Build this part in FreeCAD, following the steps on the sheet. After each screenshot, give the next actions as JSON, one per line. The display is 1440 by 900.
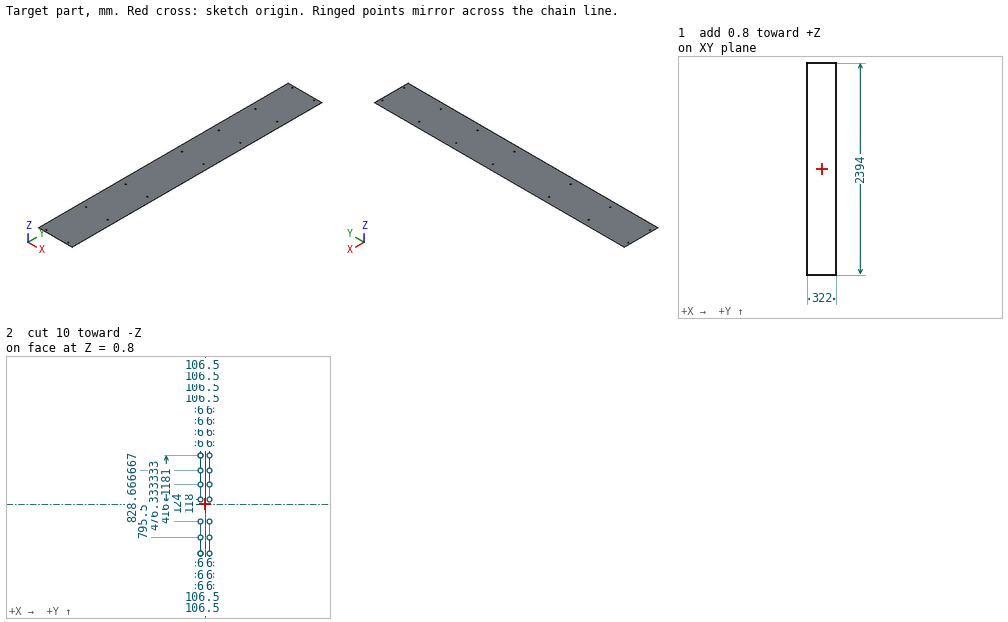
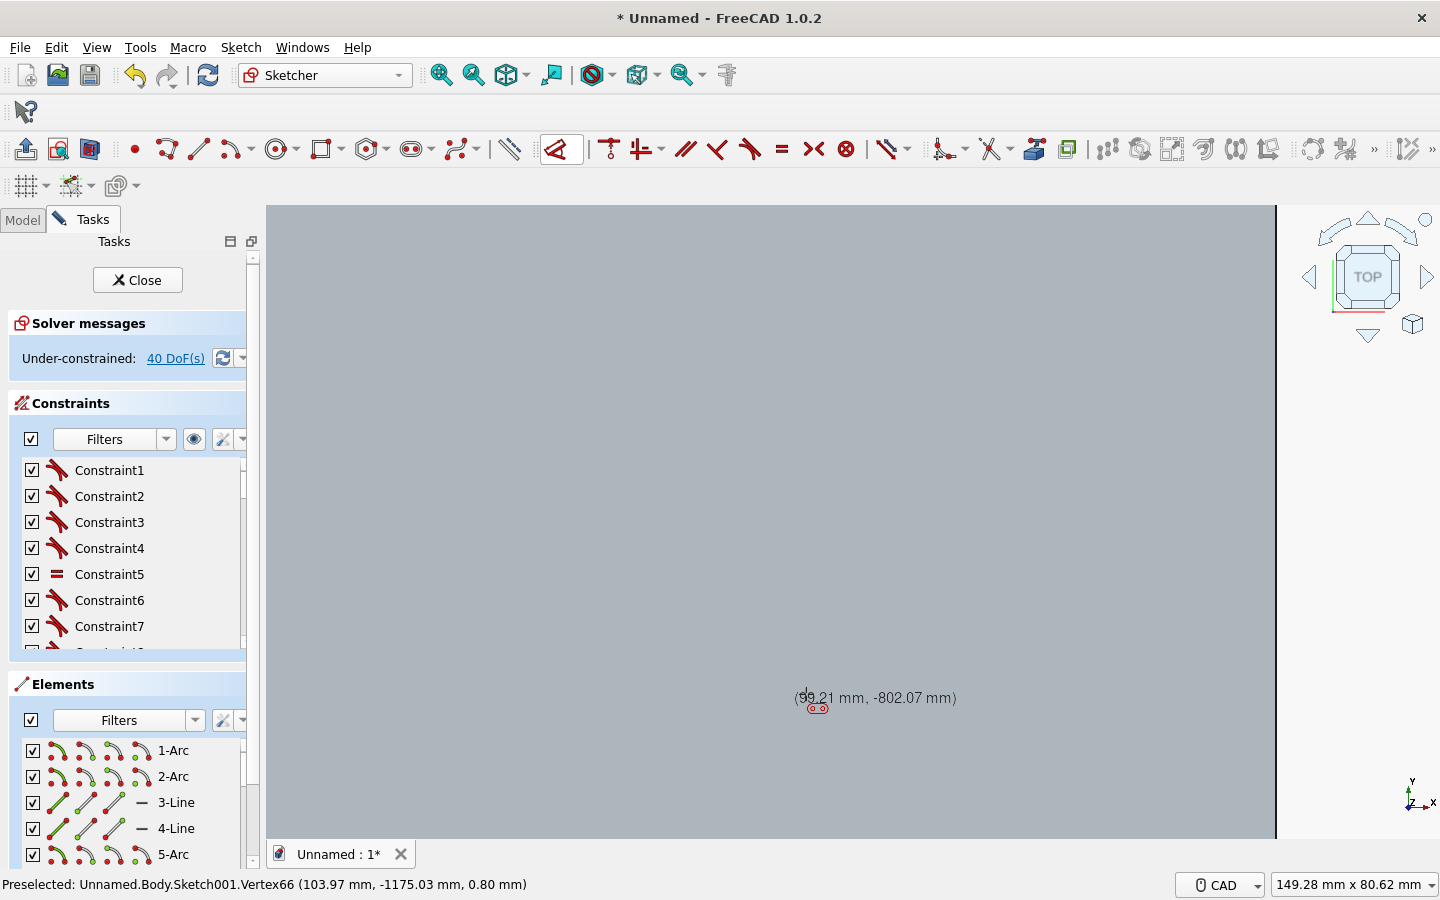
{"action": "scroll", "coordinate": [806, 694], "scroll_direction": "down", "scroll_amount": 18}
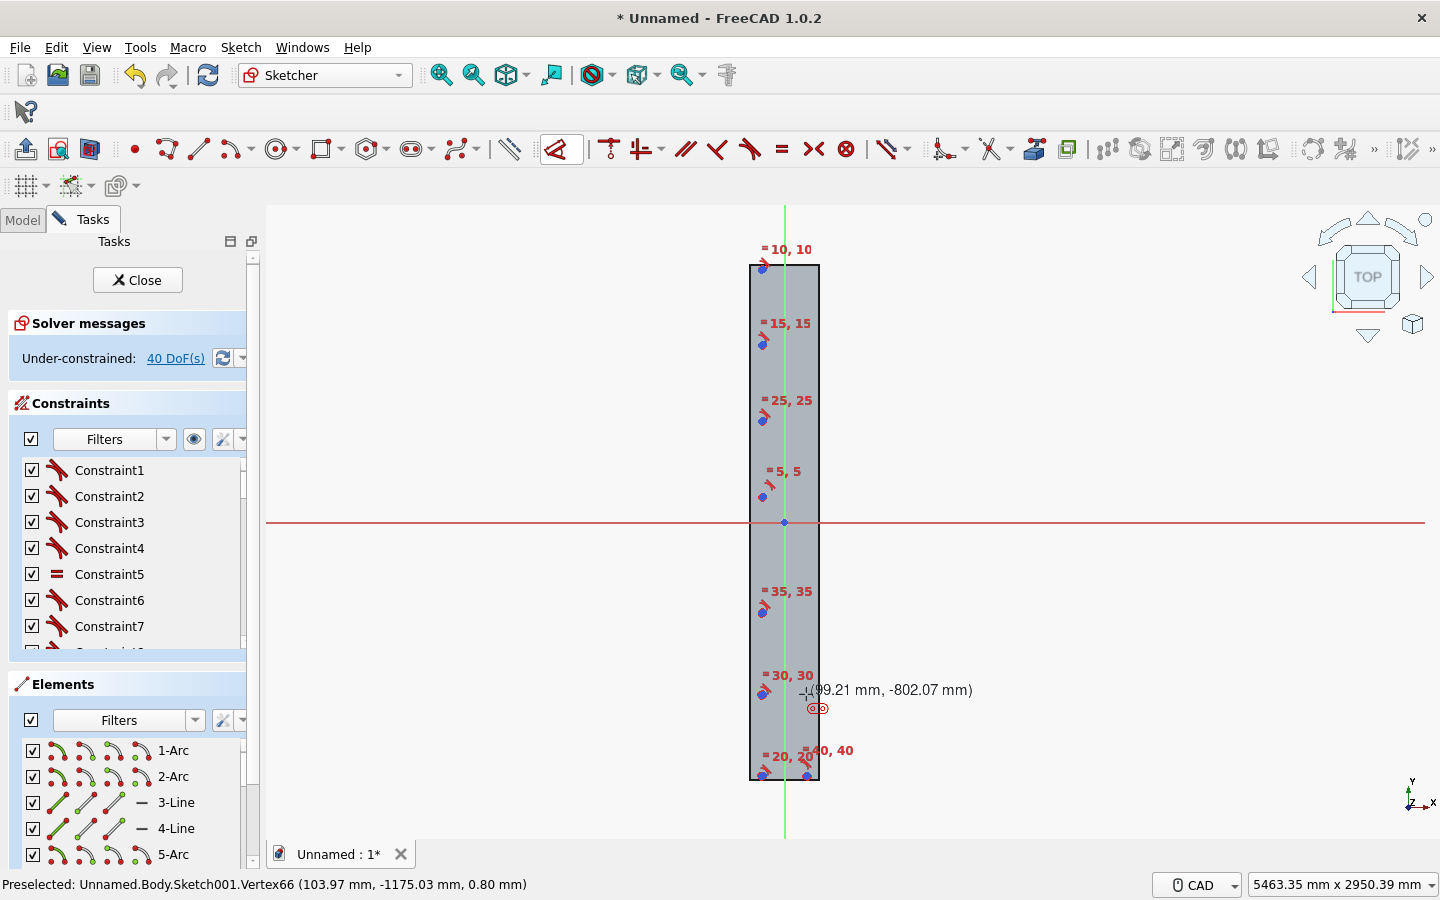
{"action": "left_click", "coordinate": [806, 694]}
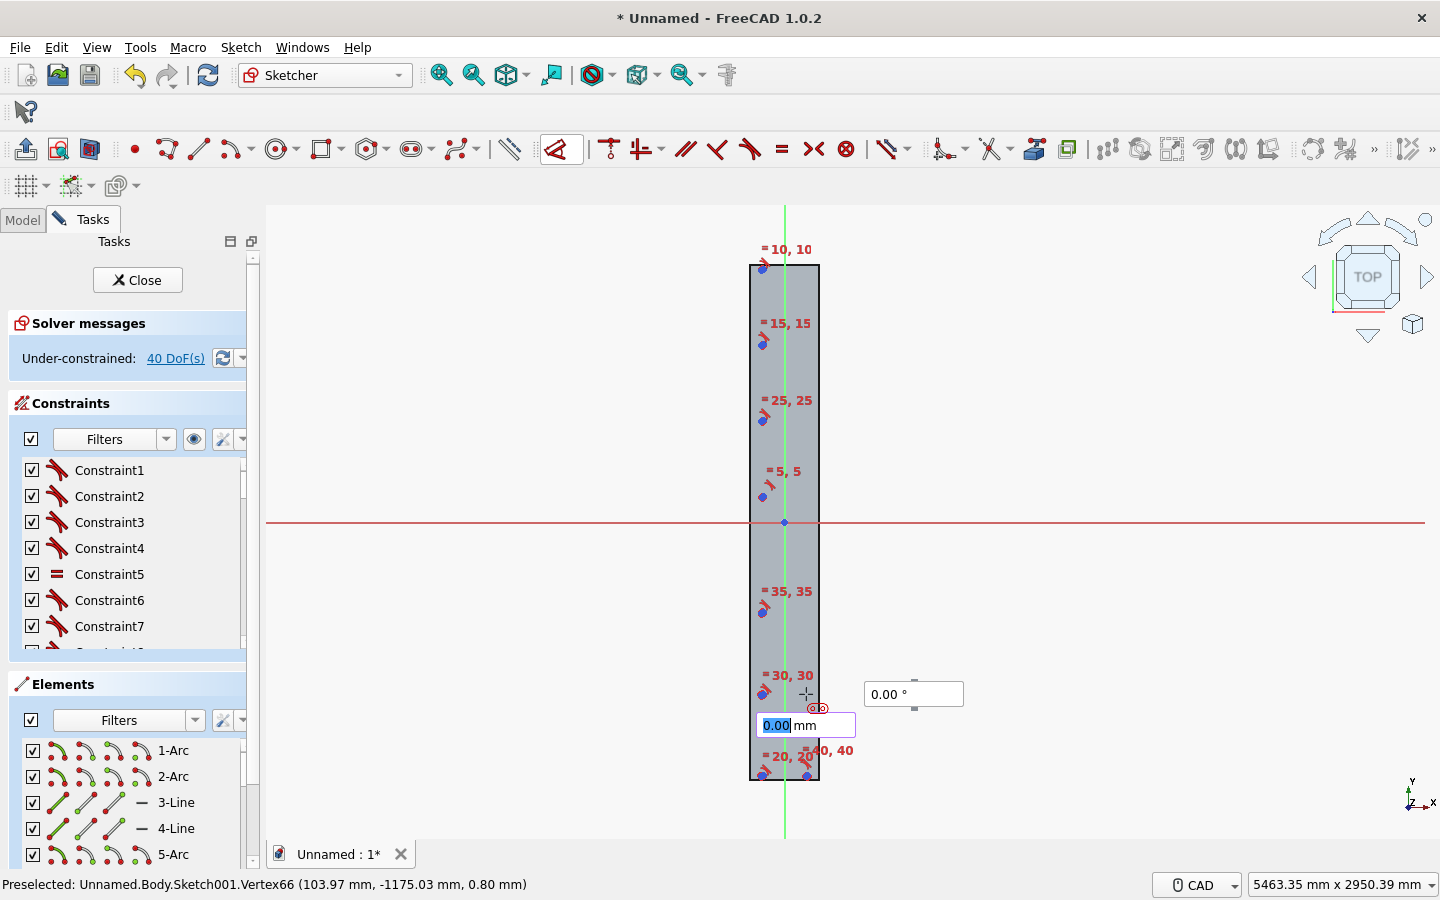
{"action": "scroll", "coordinate": [808, 694], "scroll_direction": "up", "scroll_amount": 13}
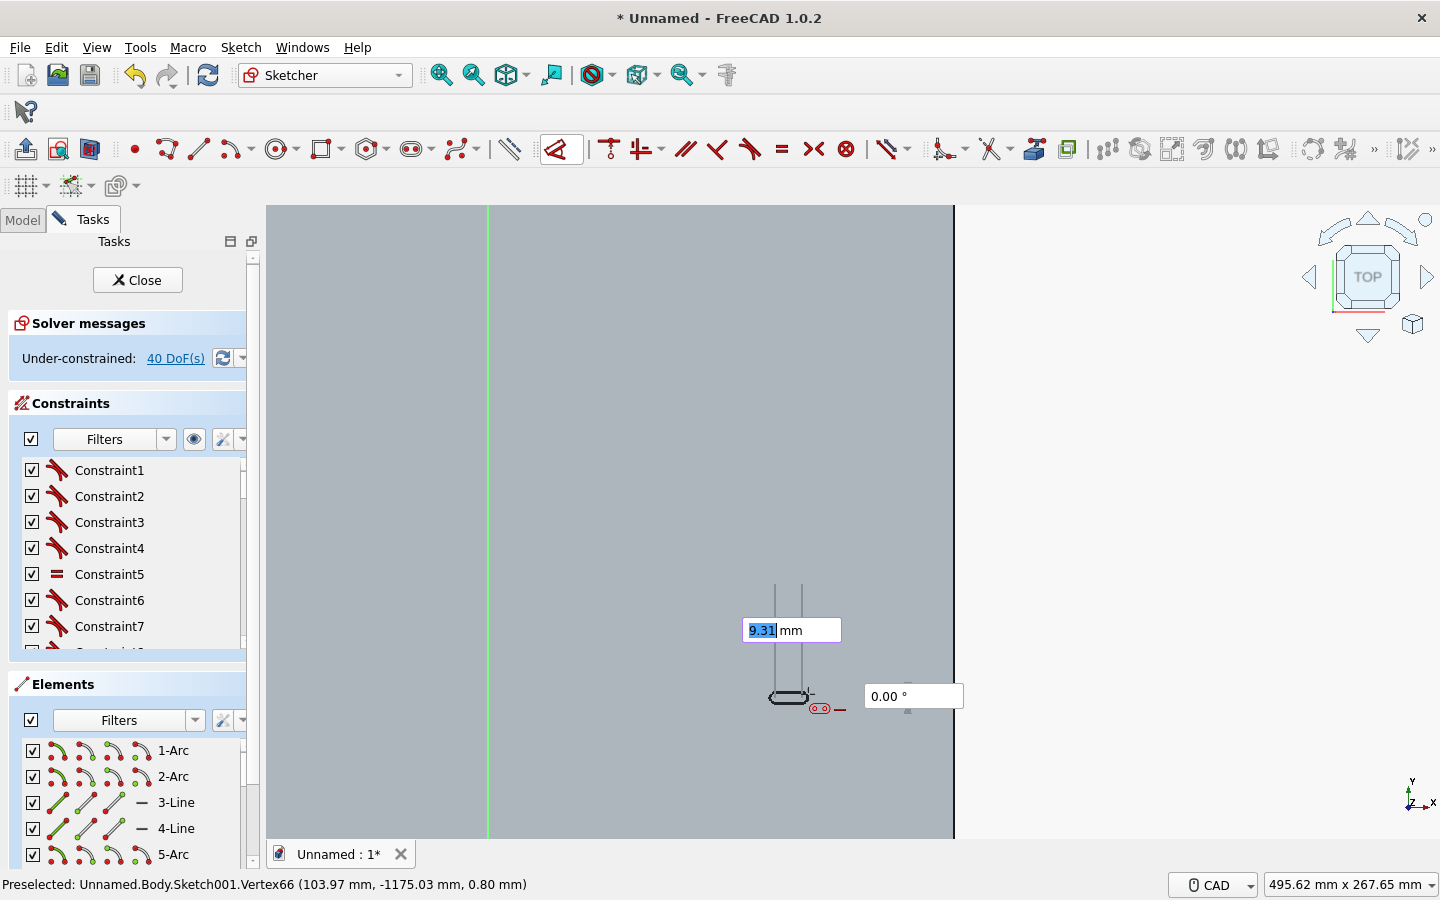
{"action": "left_click", "coordinate": [796, 684]}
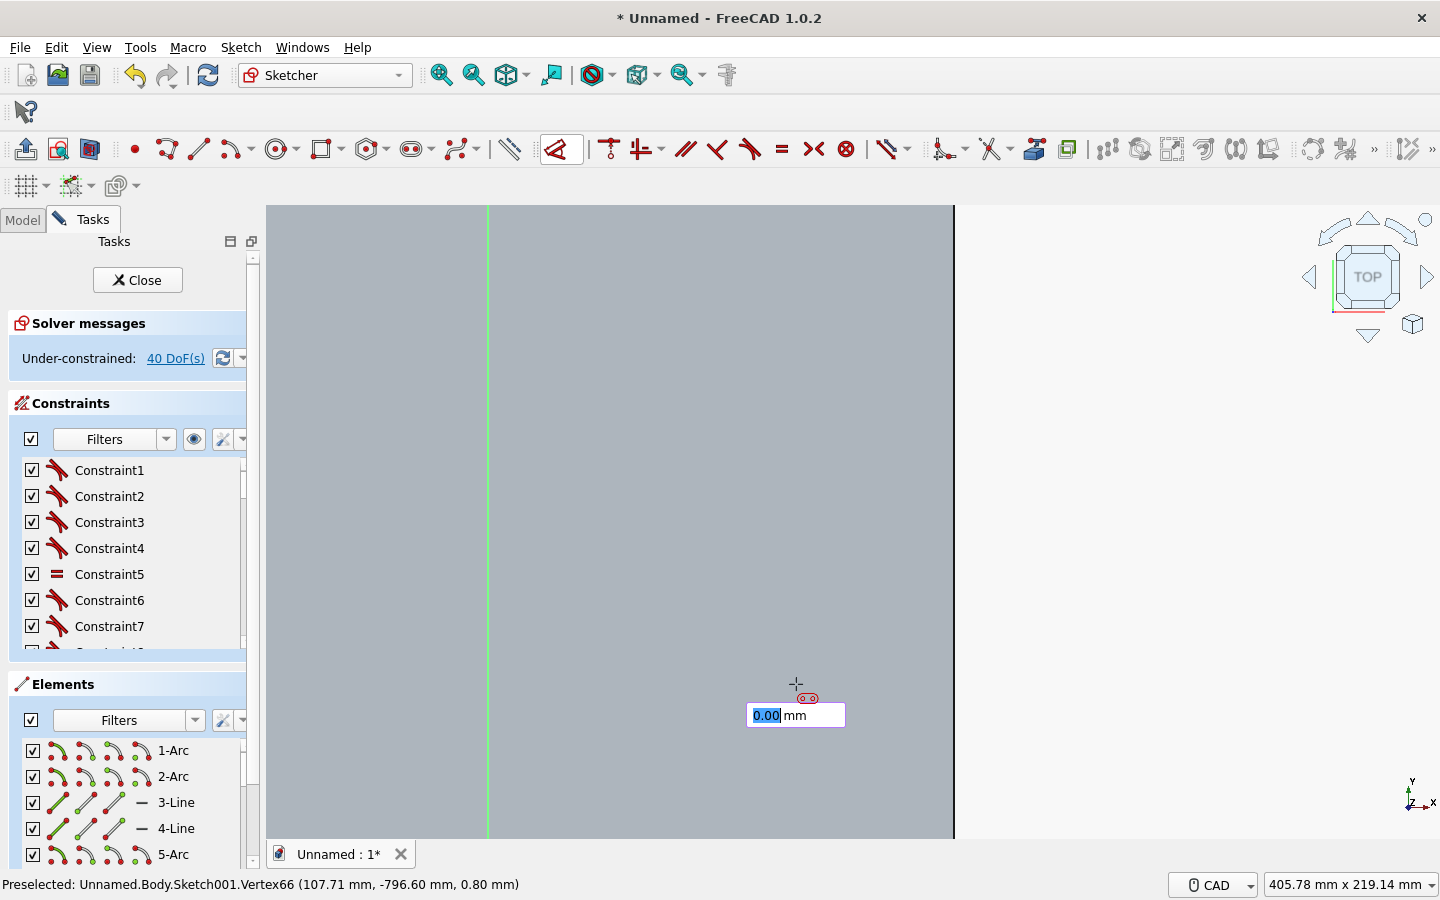
{"action": "scroll", "coordinate": [788, 679], "scroll_direction": "up", "scroll_amount": 4}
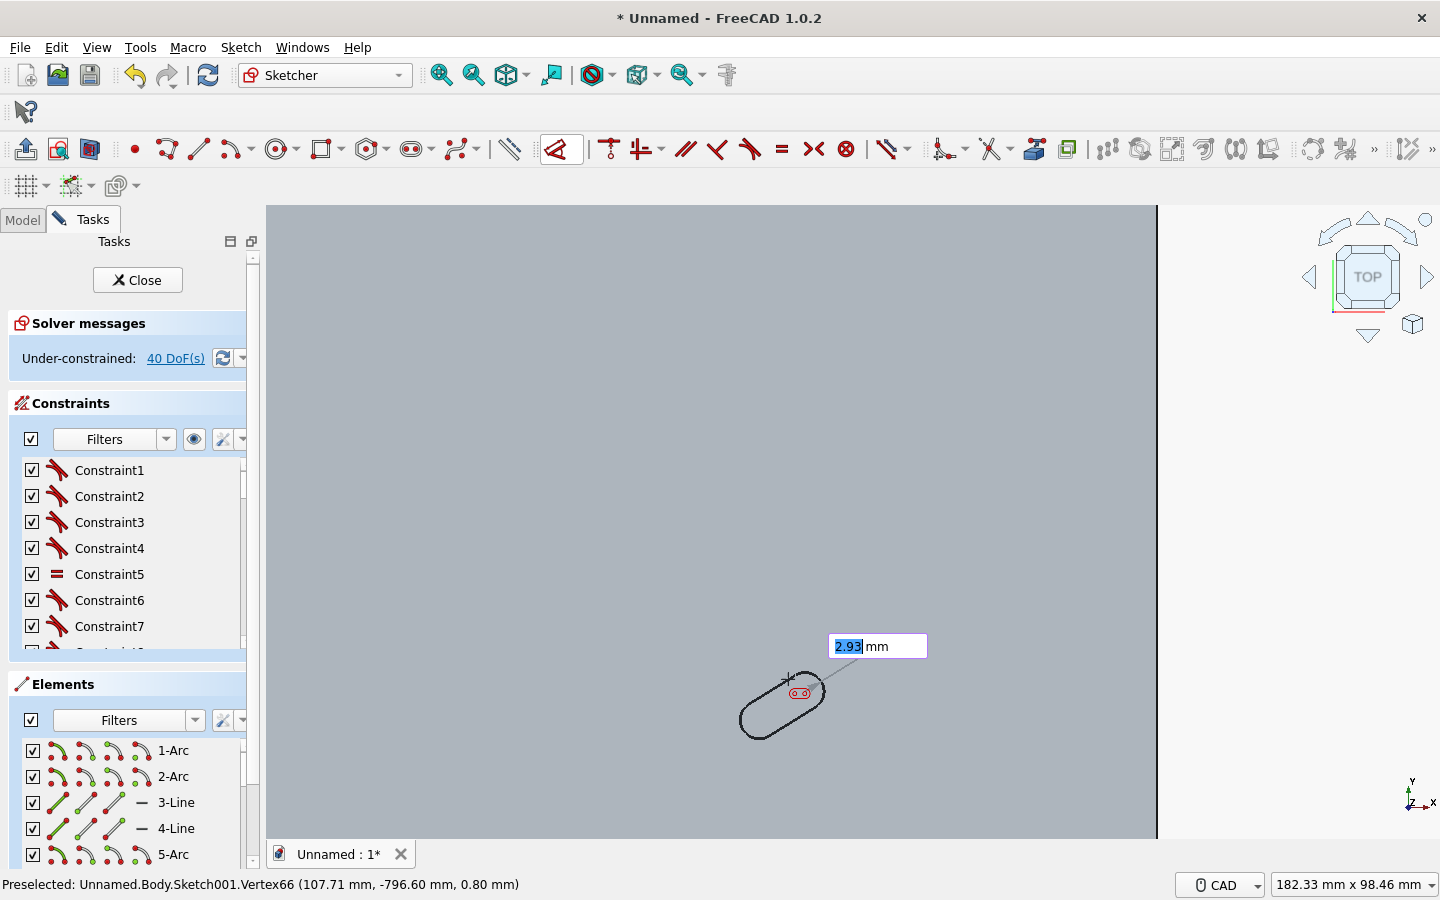
{"action": "left_click", "coordinate": [787, 678]}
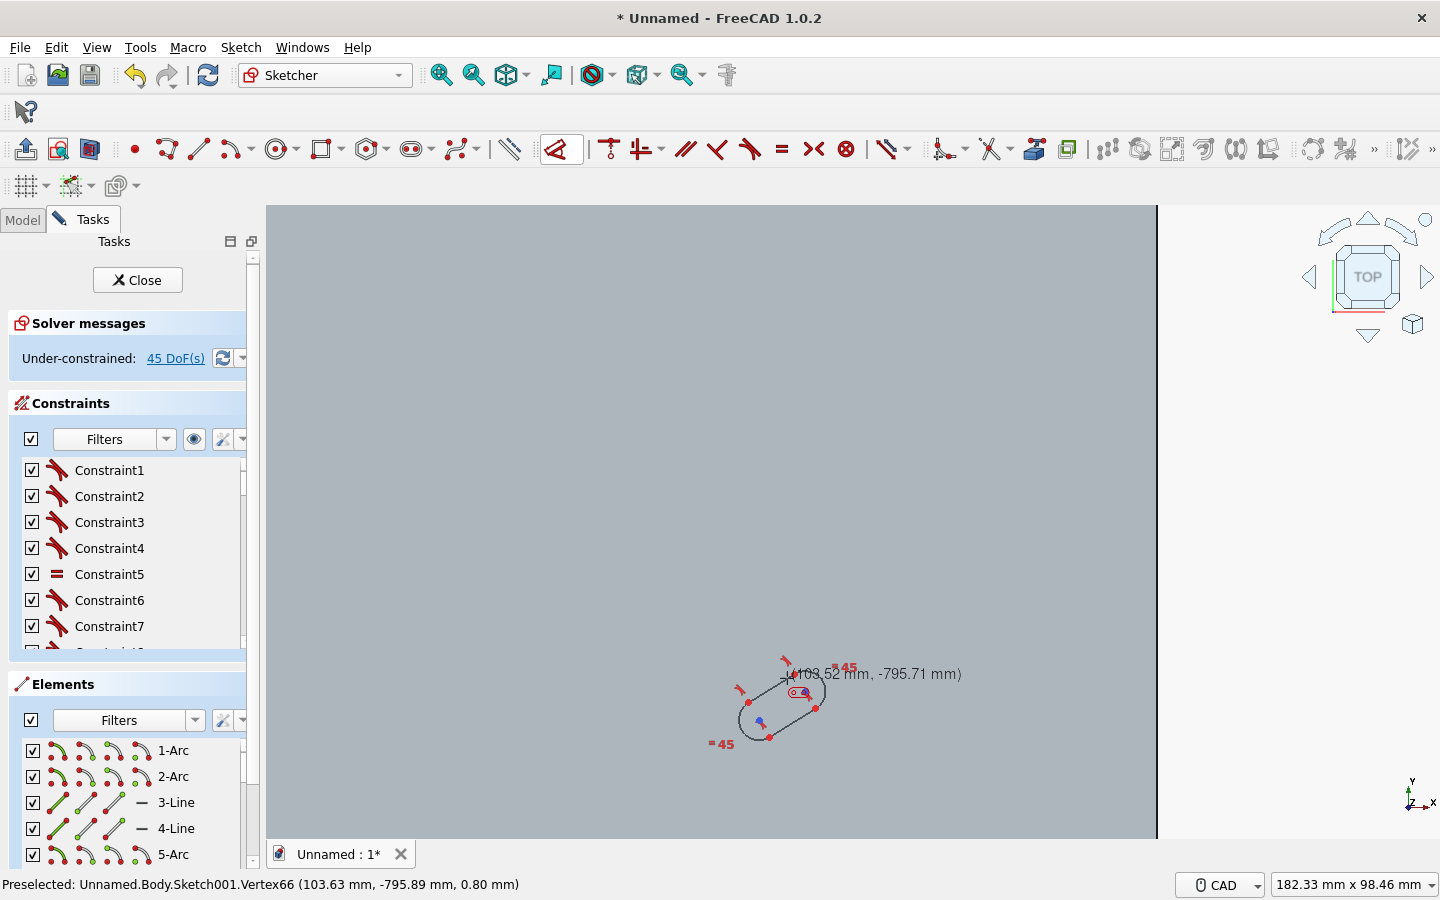
{"action": "scroll", "coordinate": [807, 693], "scroll_direction": "down", "scroll_amount": 17}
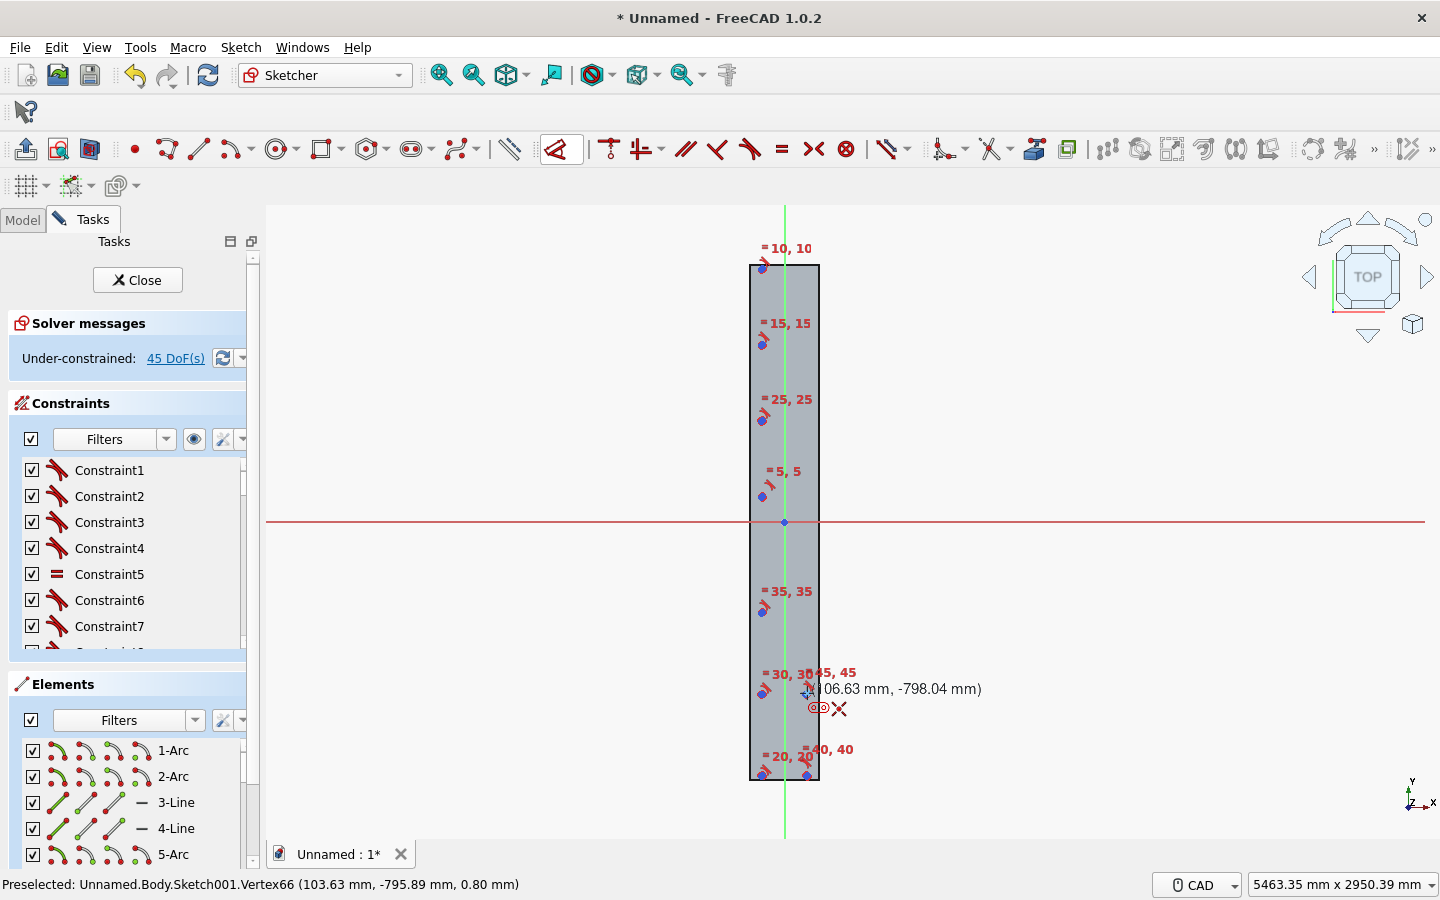
{"action": "scroll", "coordinate": [806, 612], "scroll_direction": "up", "scroll_amount": 18}